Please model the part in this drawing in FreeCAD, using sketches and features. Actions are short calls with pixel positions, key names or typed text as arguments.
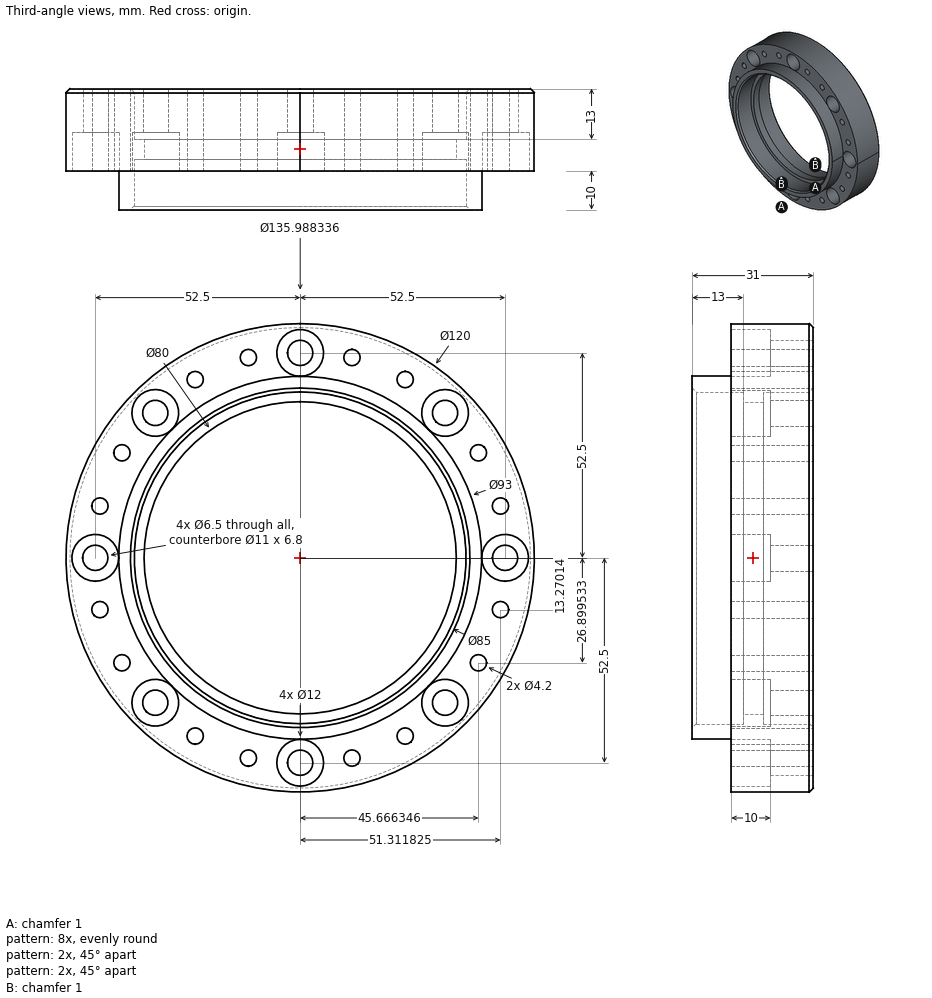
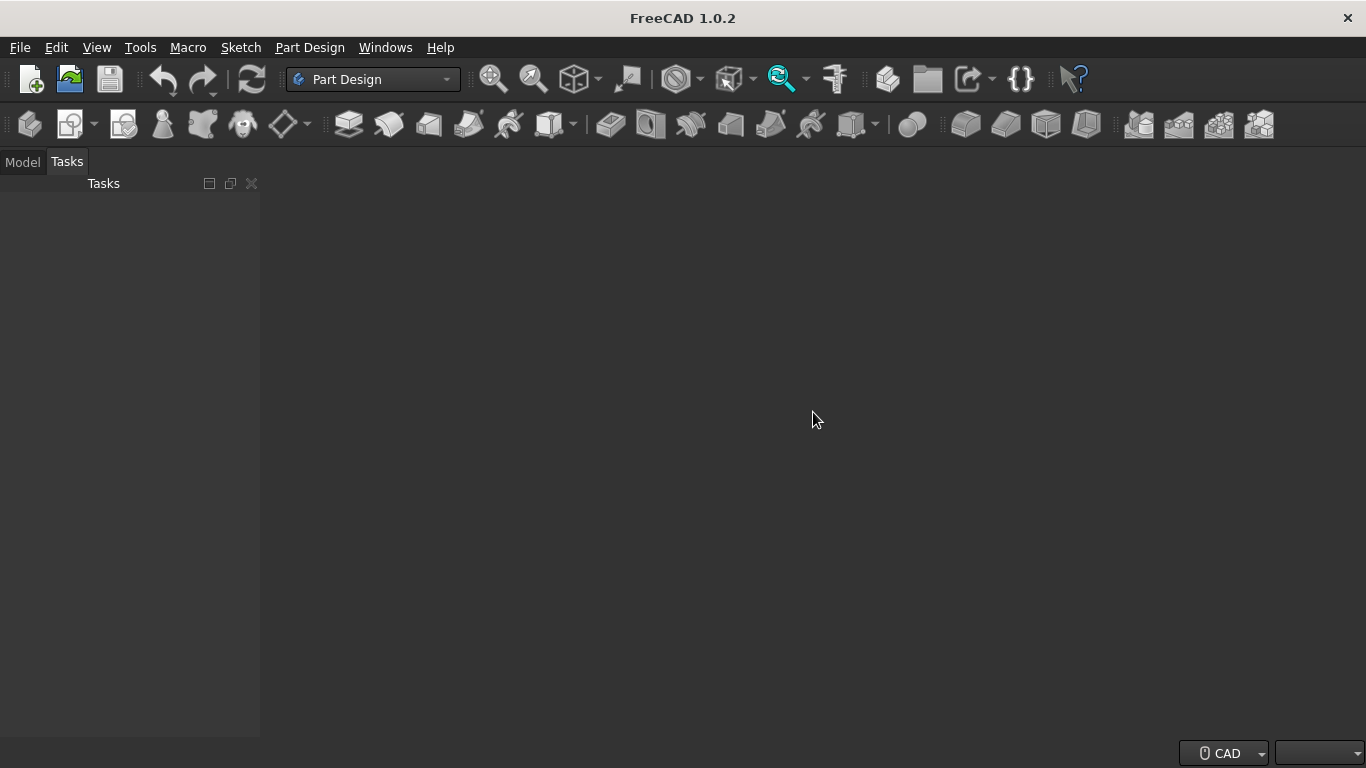
click(30, 80)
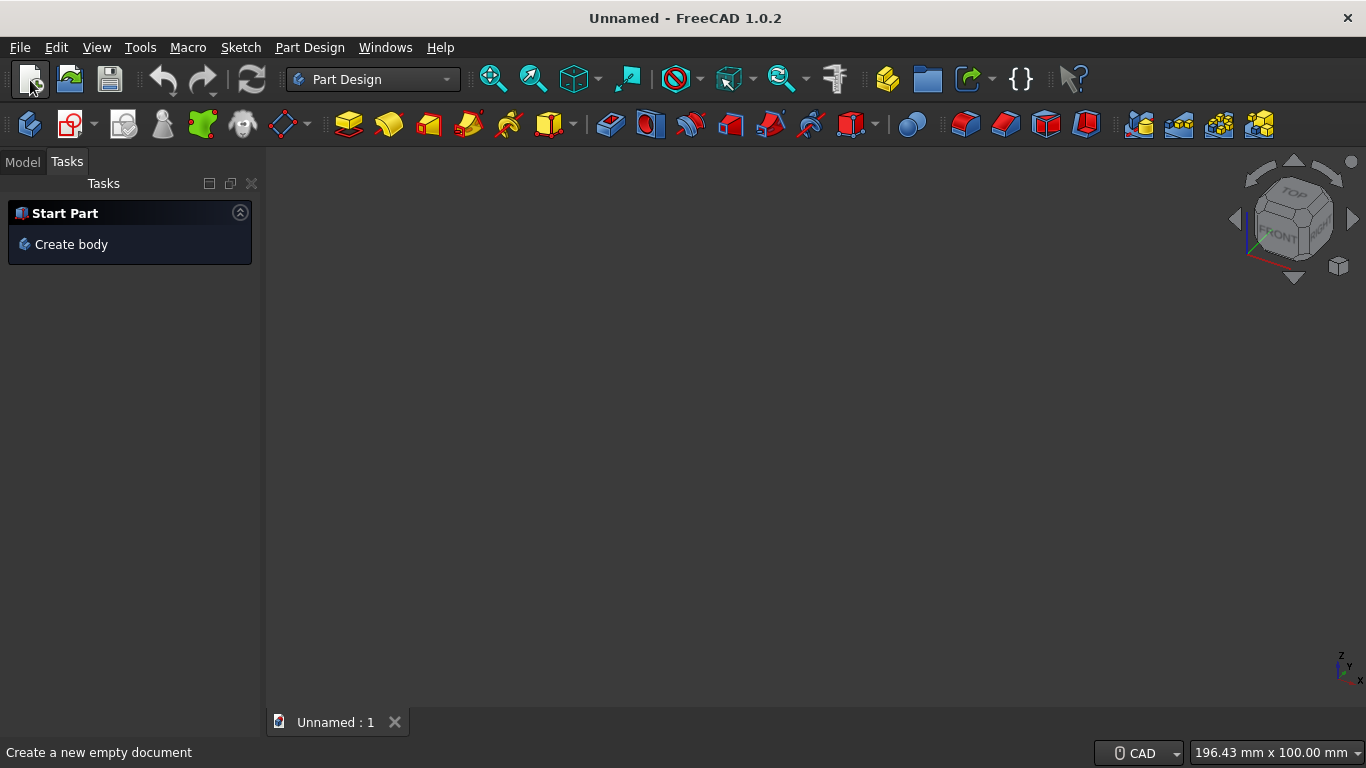
click(70, 124)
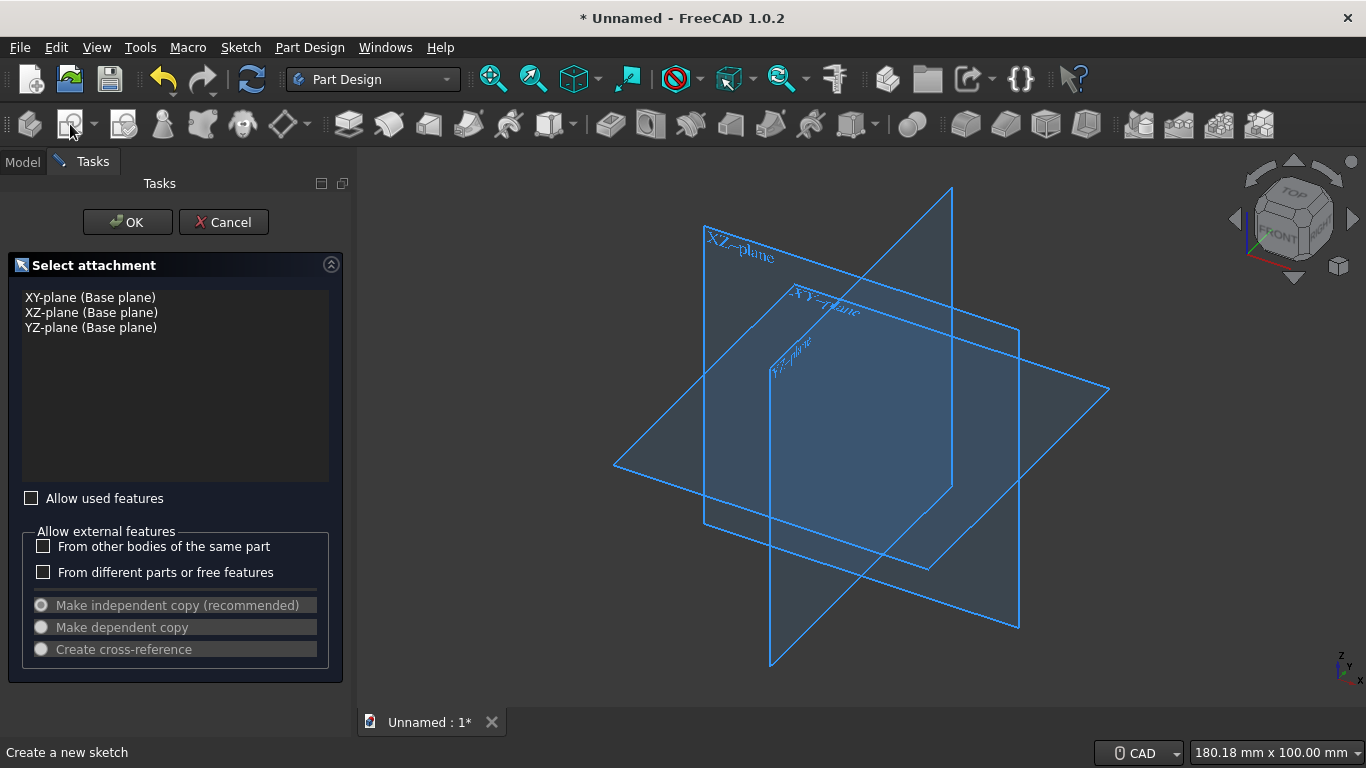
click(82, 312)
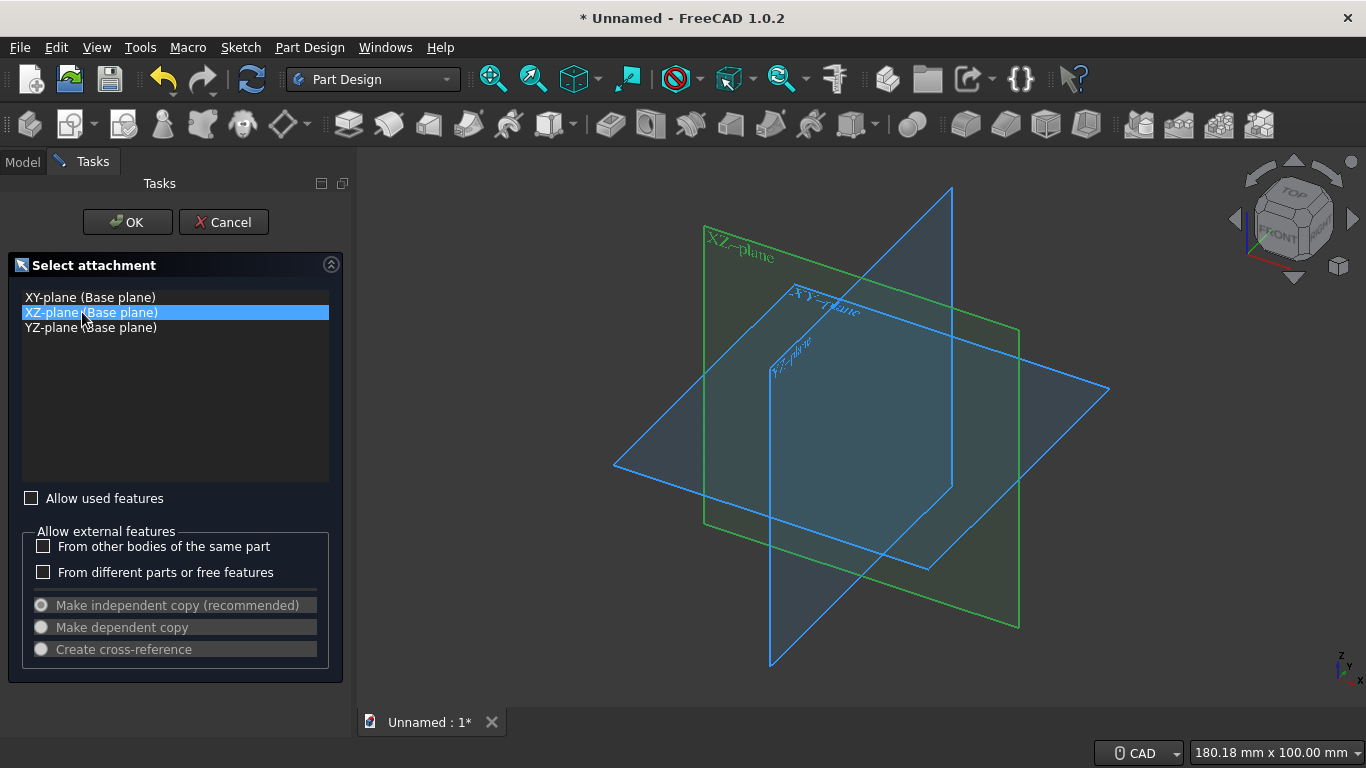
click(128, 222)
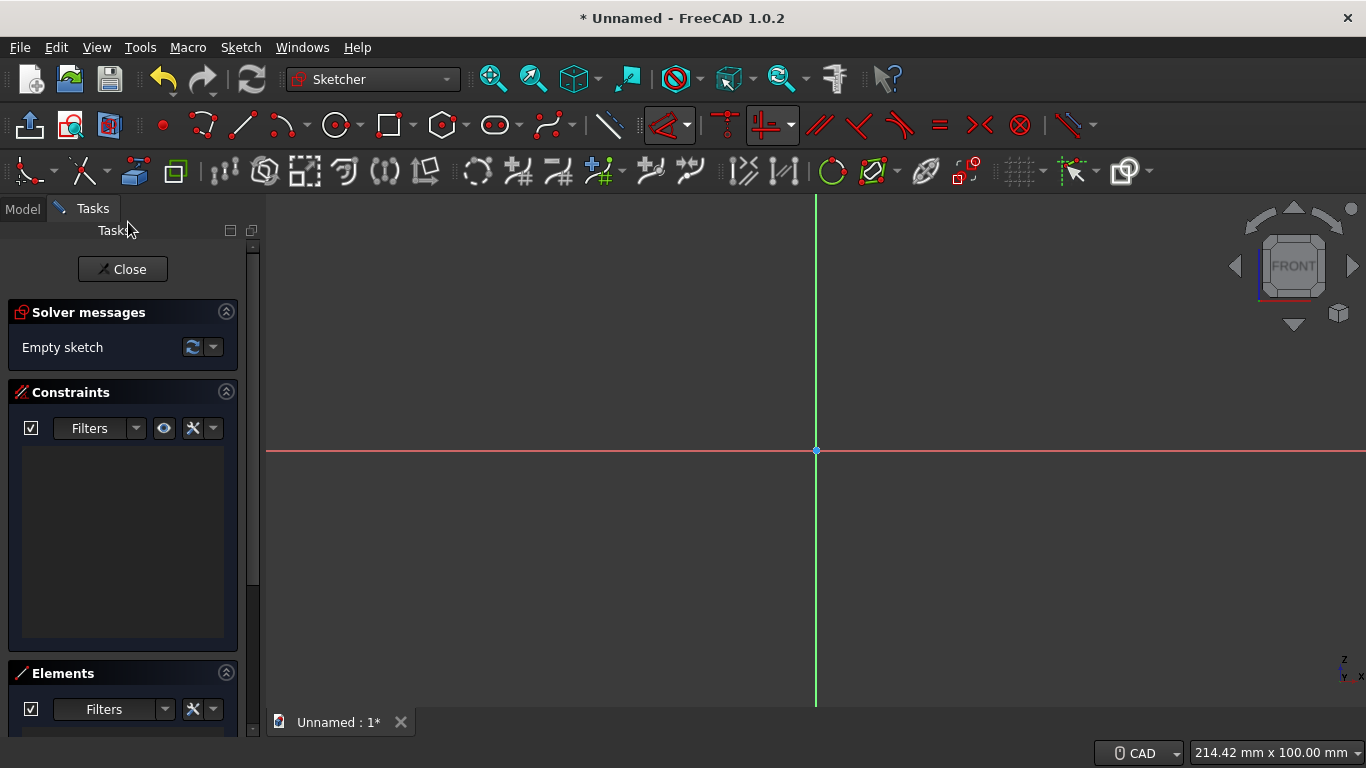
scroll(664, 451, down, 3)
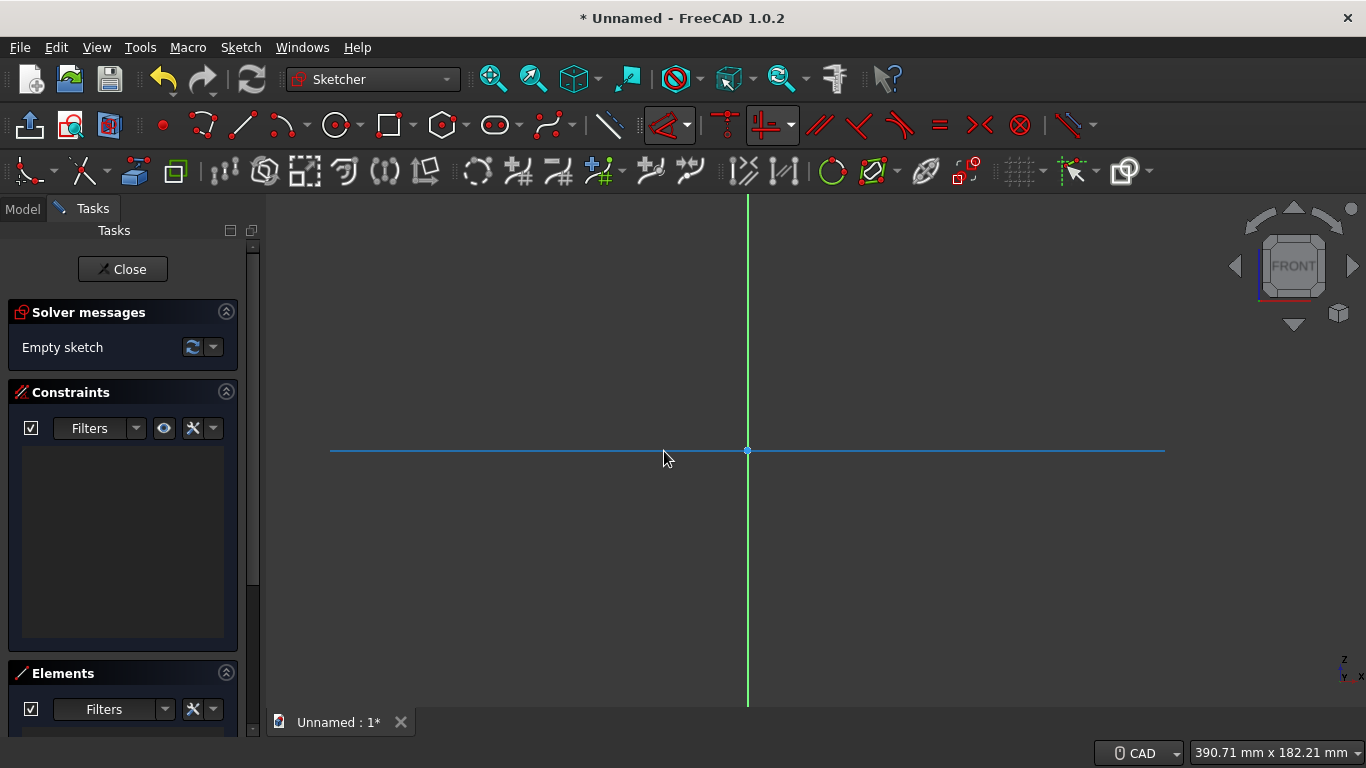
click(336, 126)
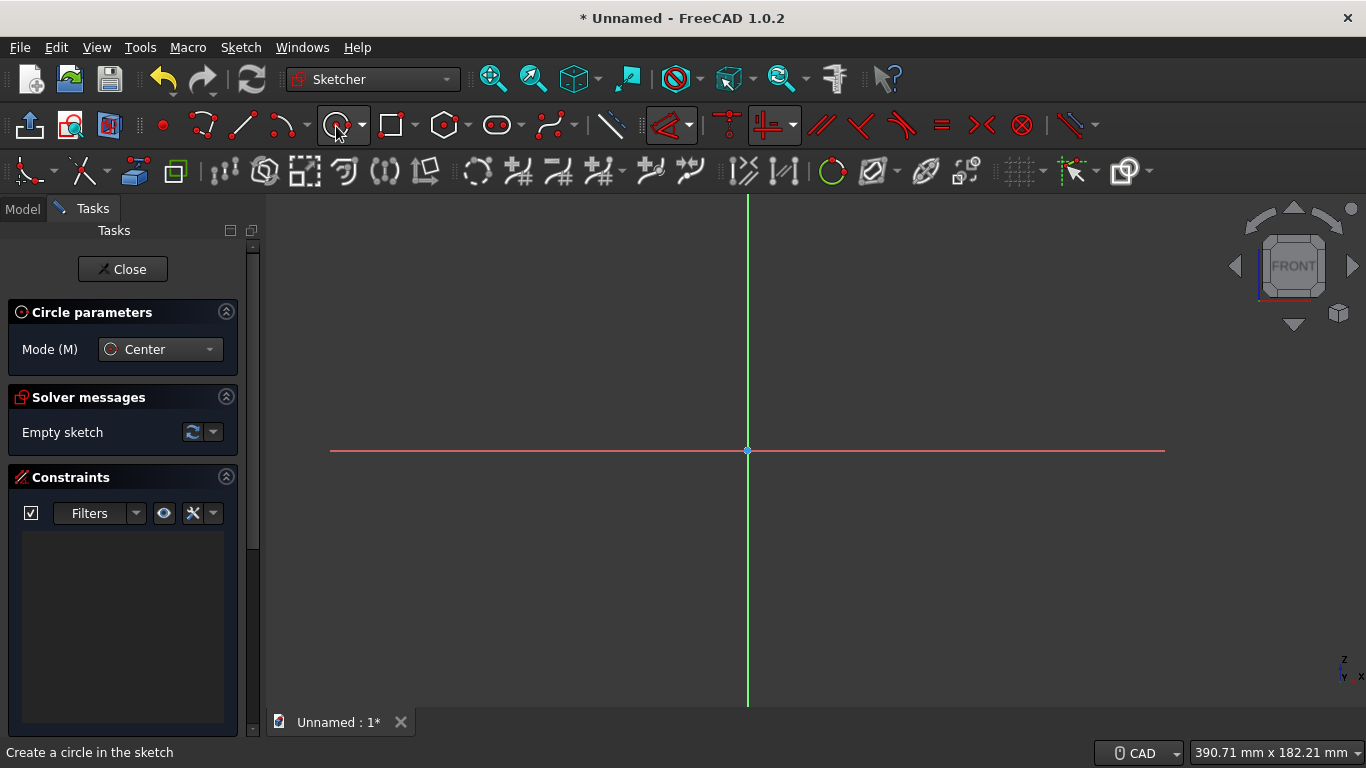
click(748, 451)
move(867, 332)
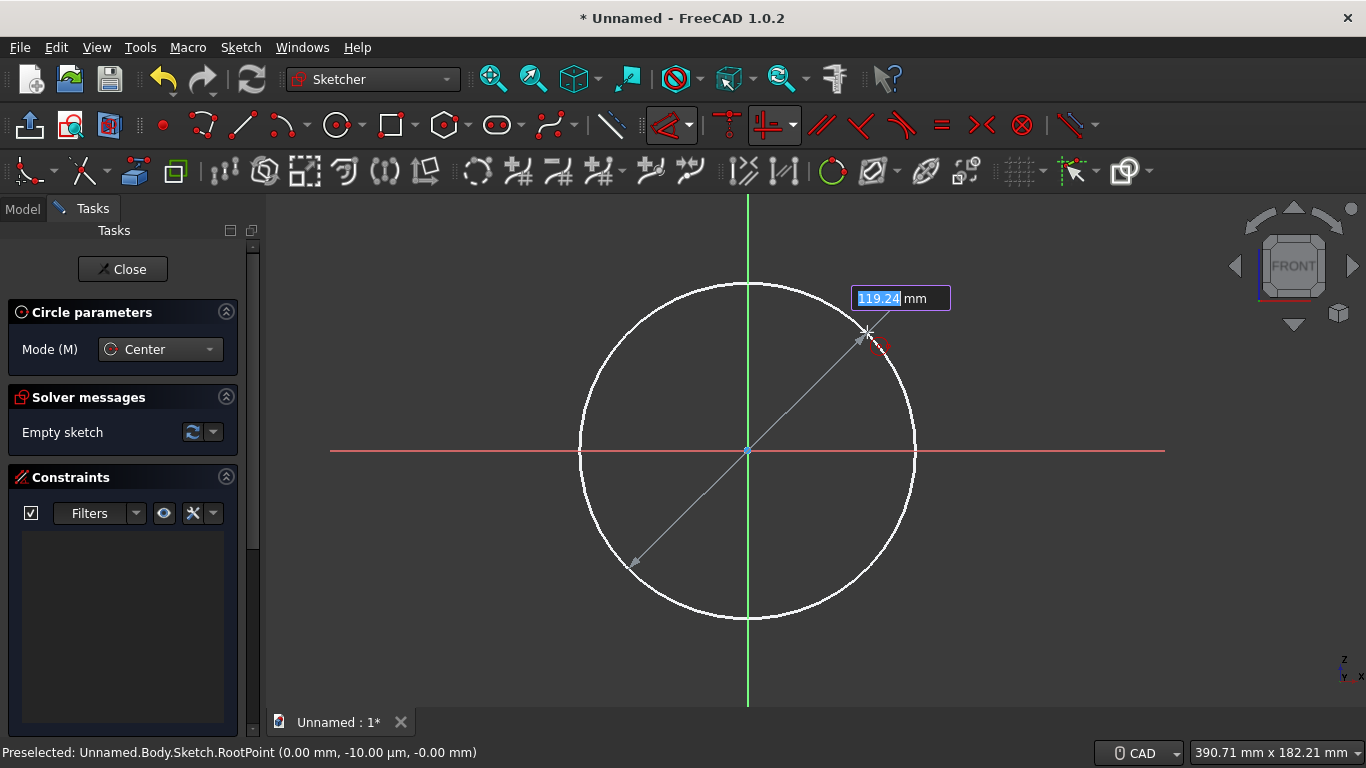
text(120)
key(Return)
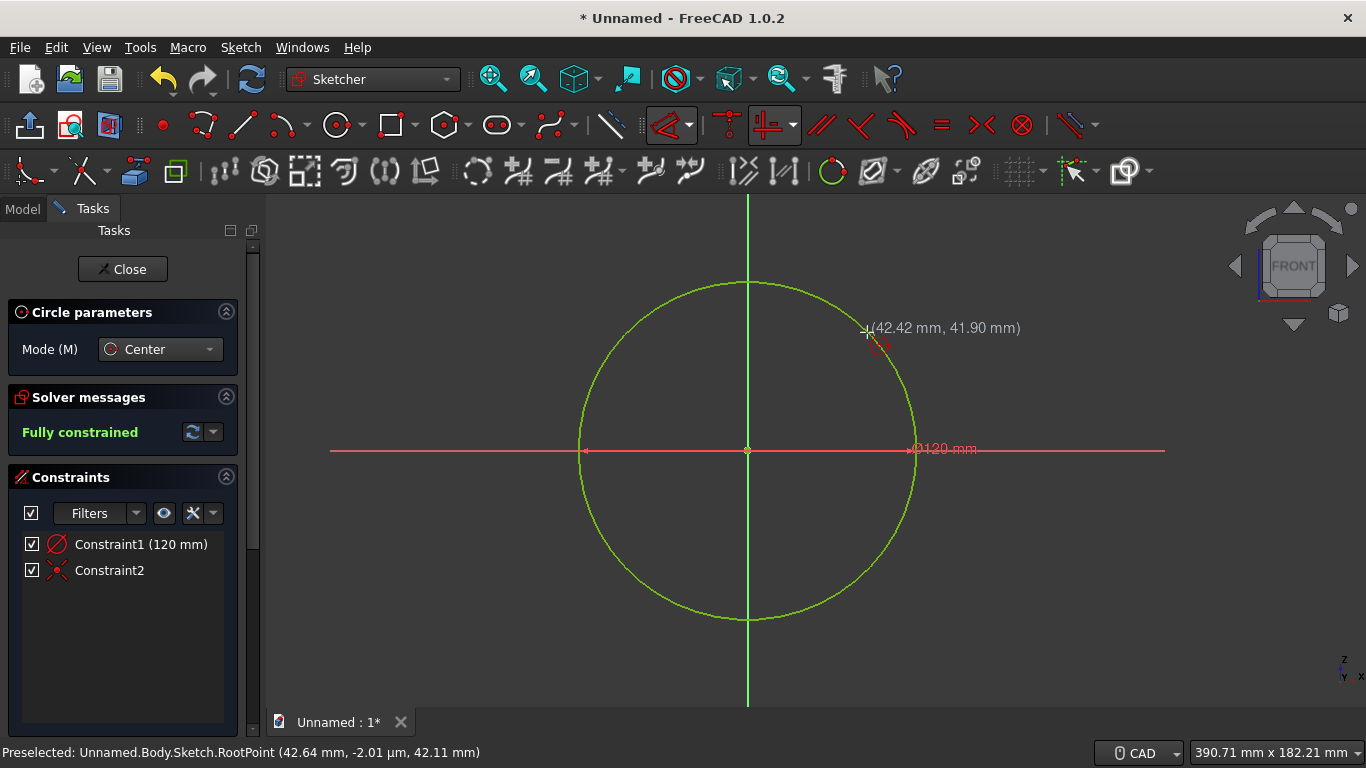
click(748, 451)
move(827, 371)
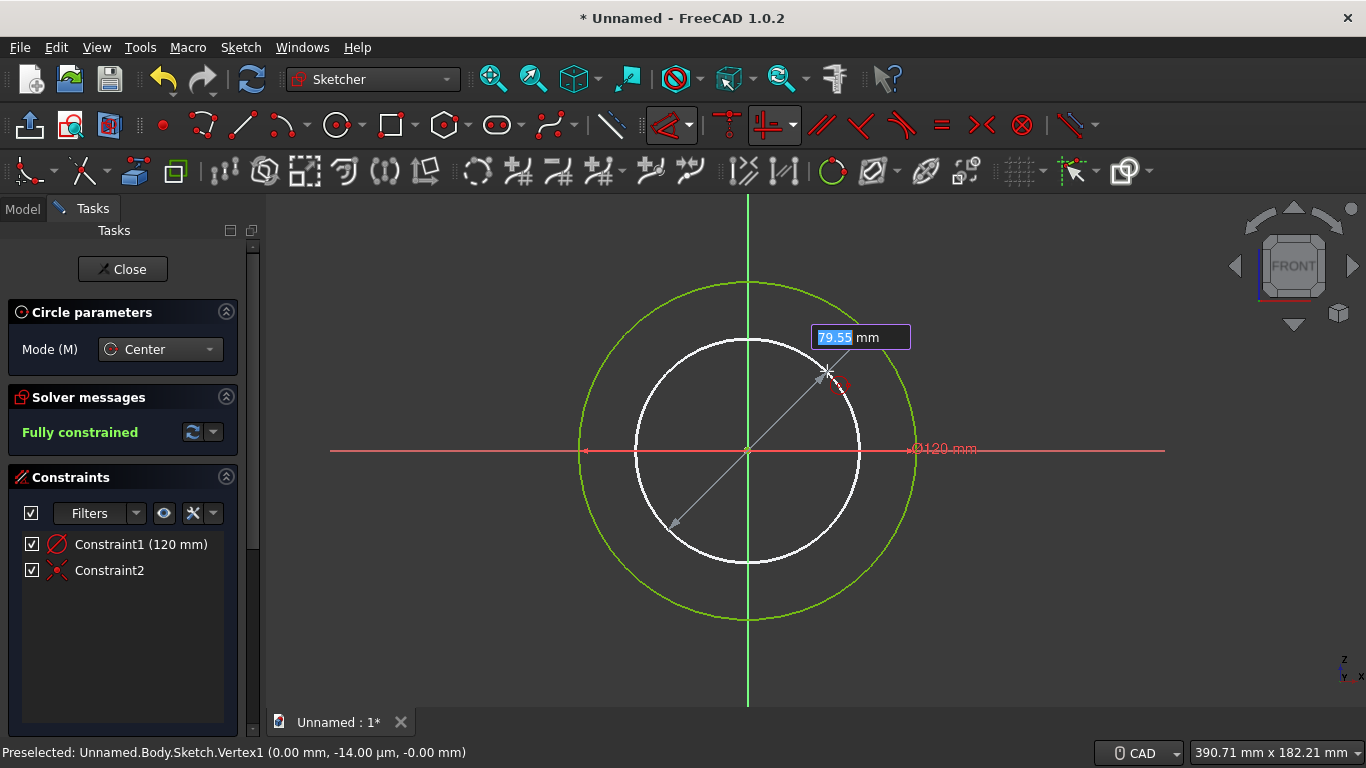
text(80)
key(Return)
key(Escape)